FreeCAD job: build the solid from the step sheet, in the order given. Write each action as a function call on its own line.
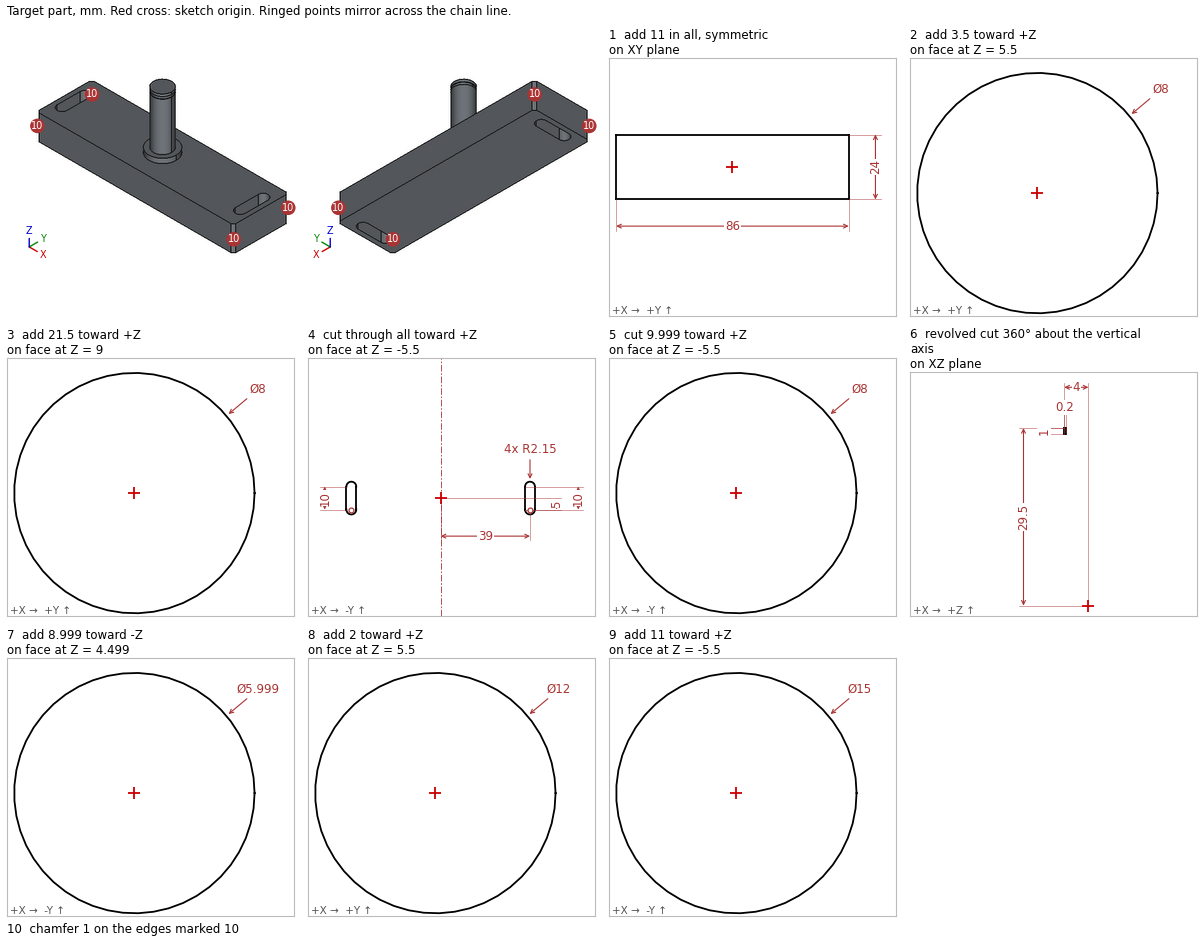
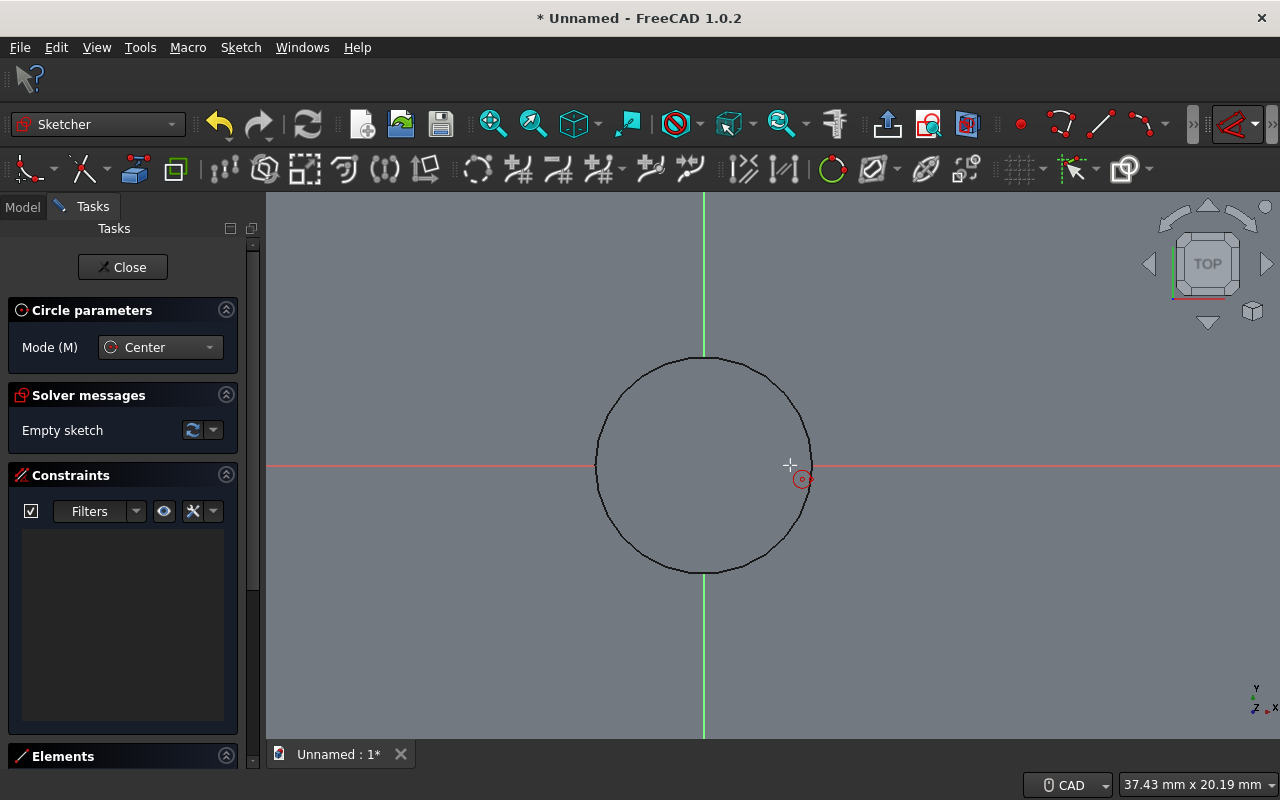
click(704, 465)
move(819, 351)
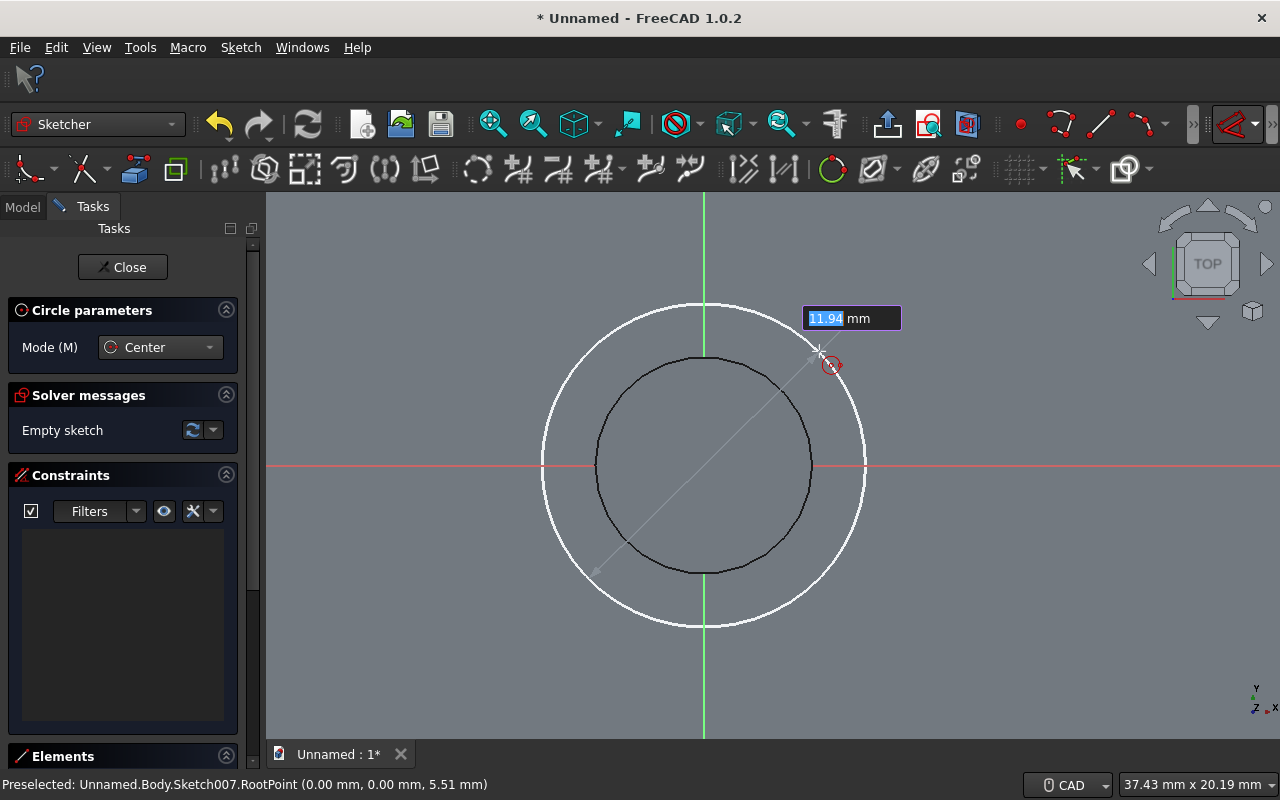
text(12)
key(Return)
key(Escape)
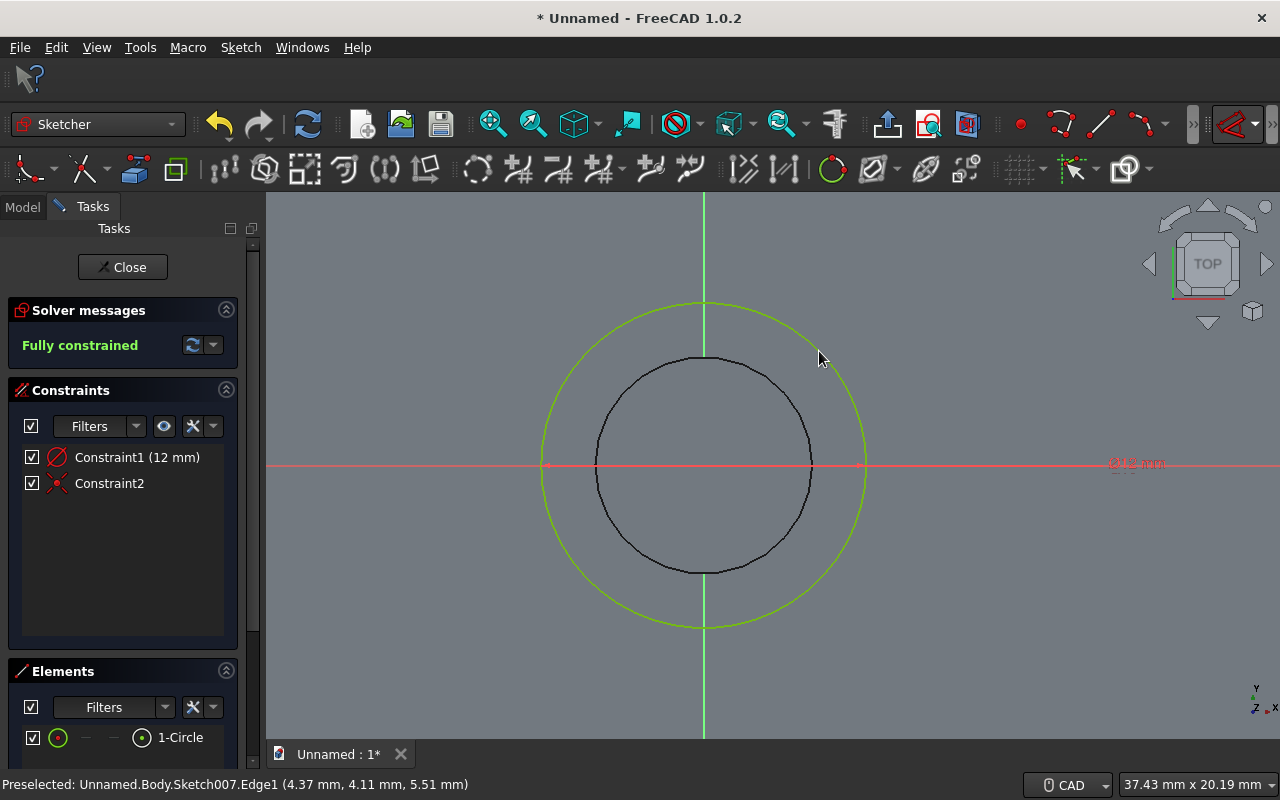
click(123, 267)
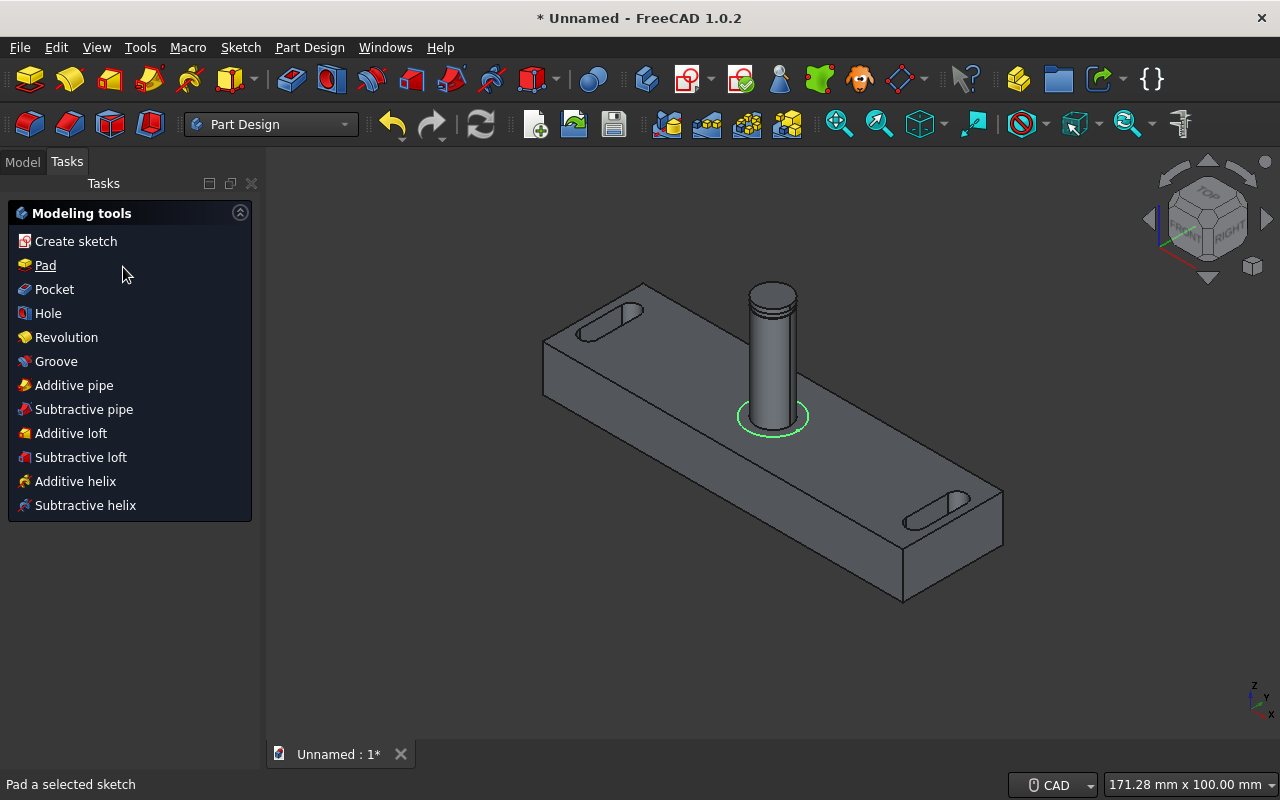
click(30, 80)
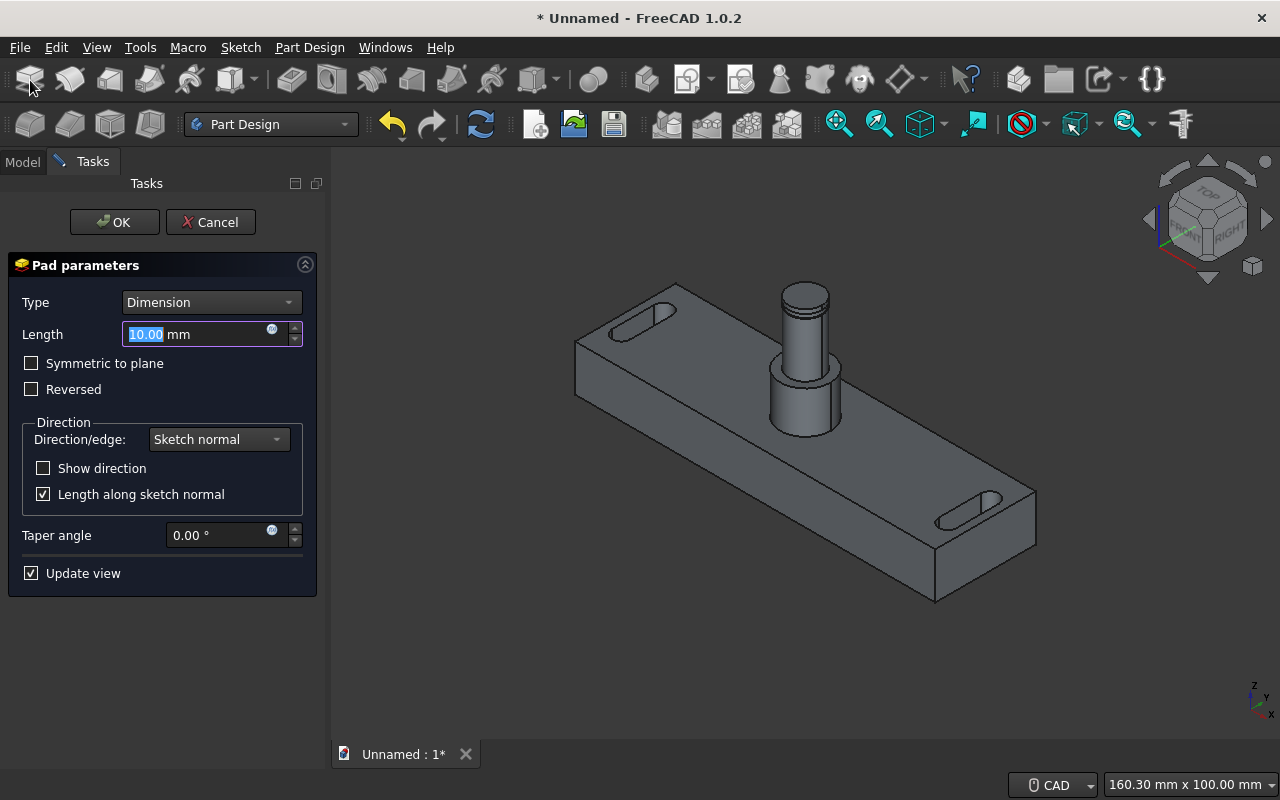
text(2)
key(Tab)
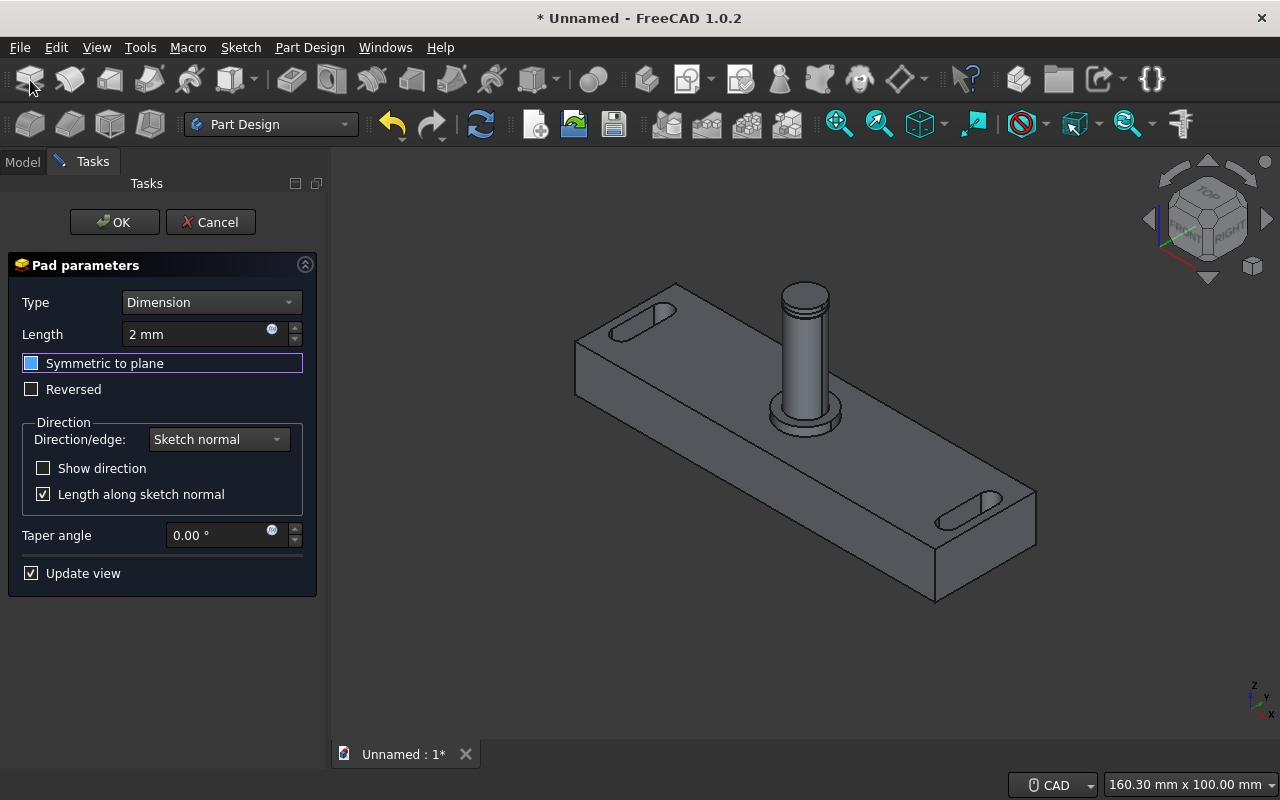
click(115, 222)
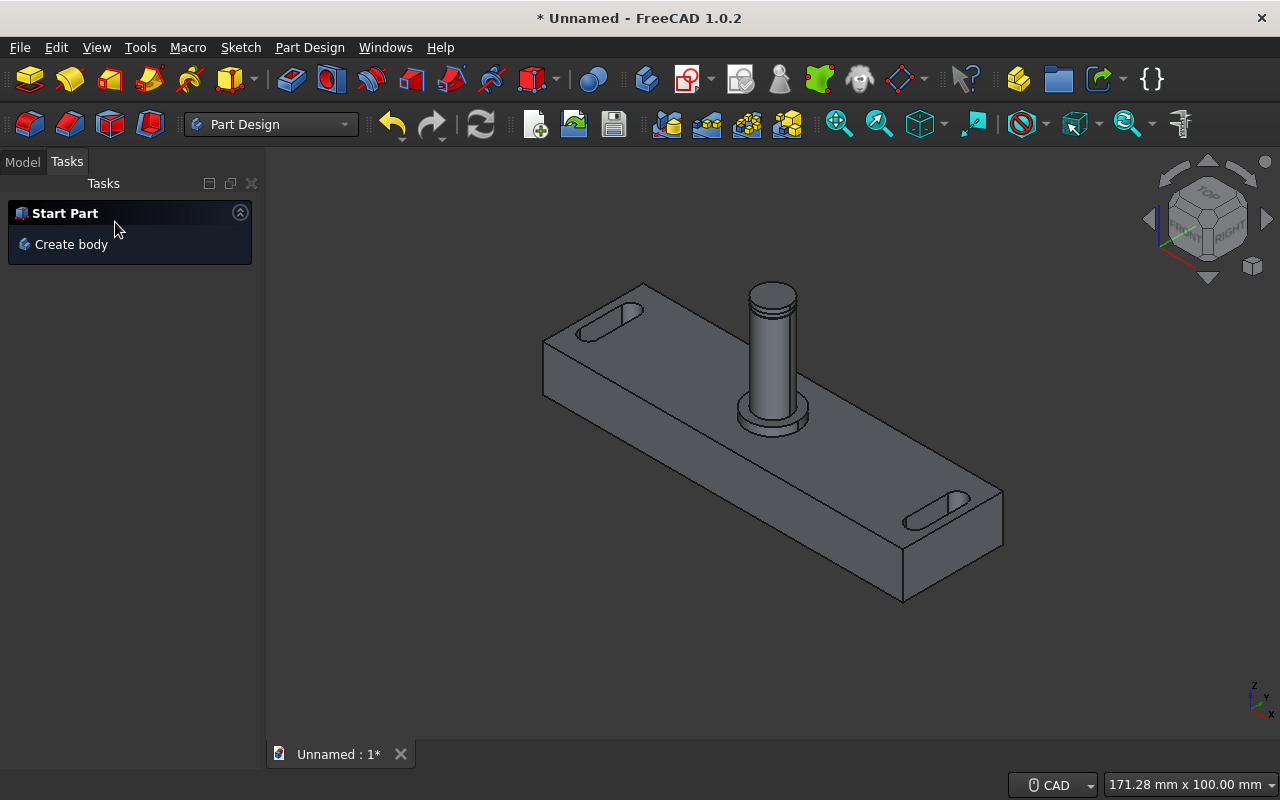
key(5)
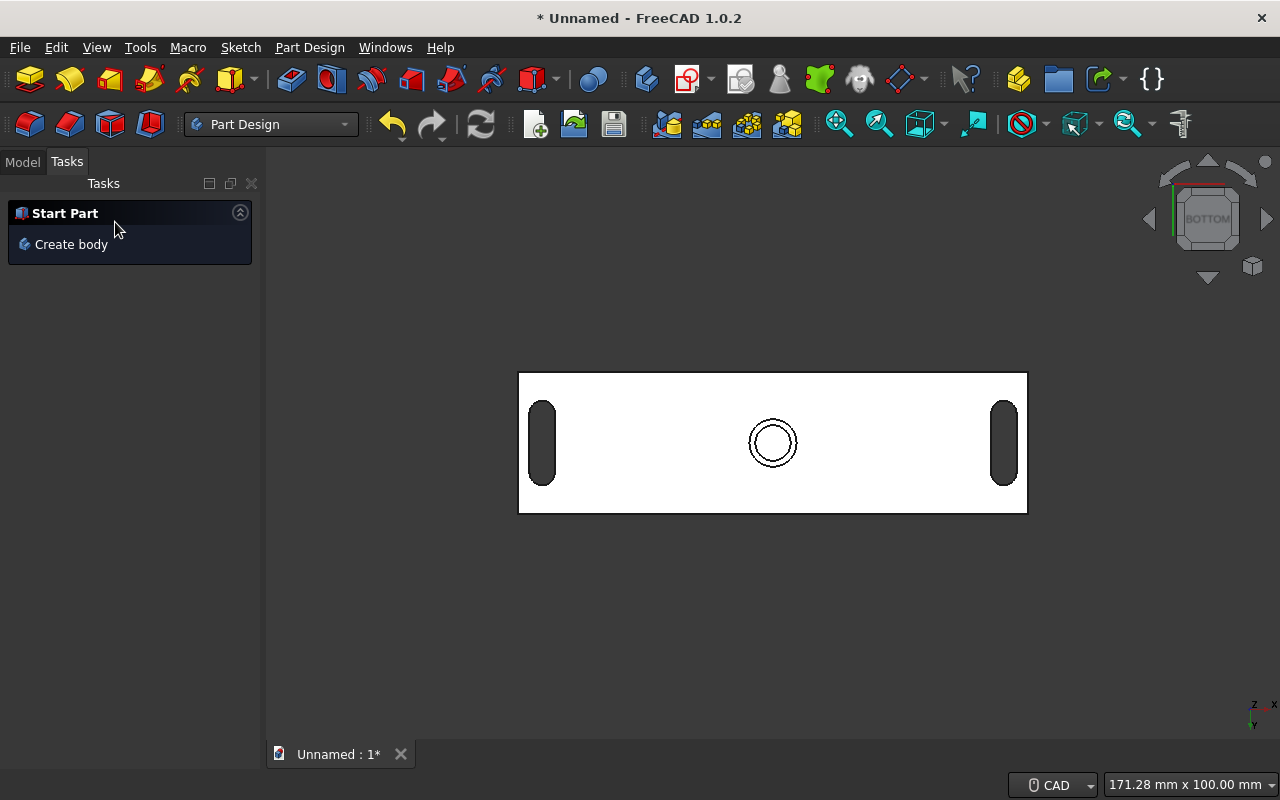
click(918, 442)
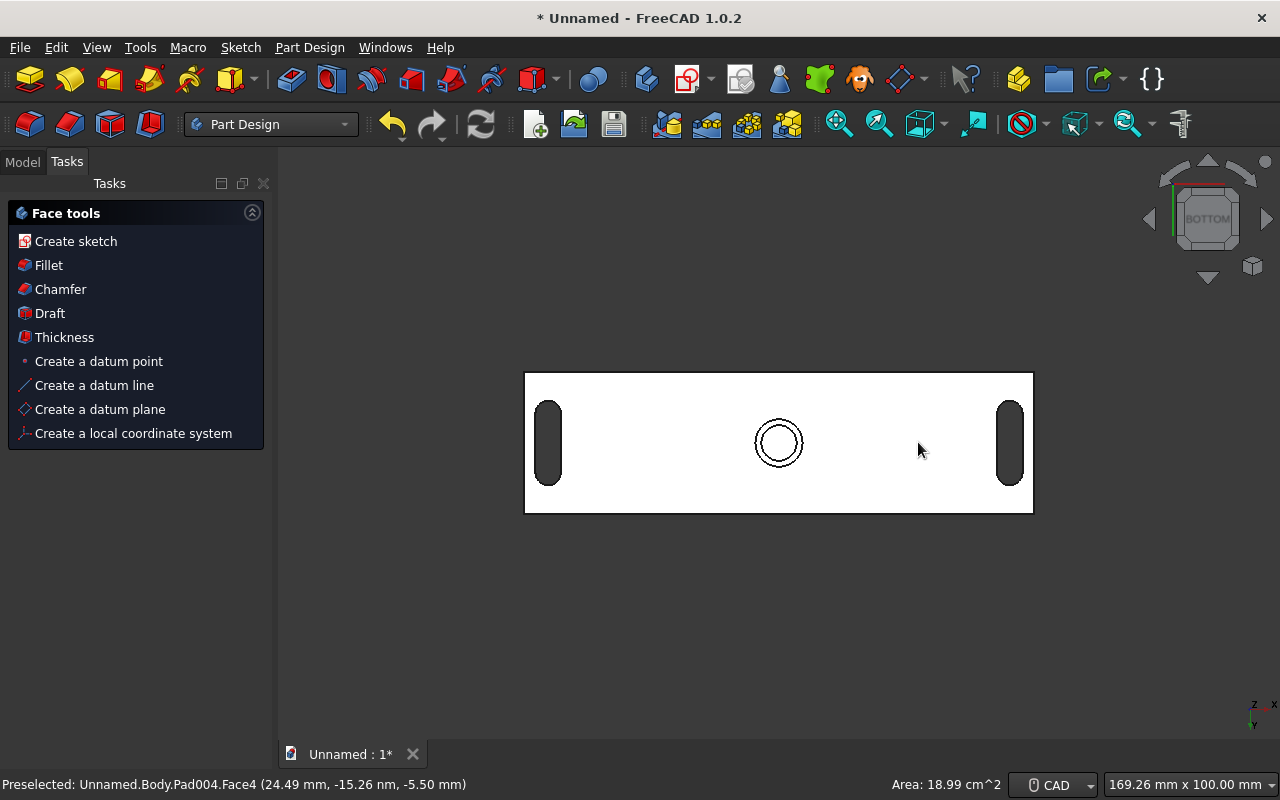
click(688, 80)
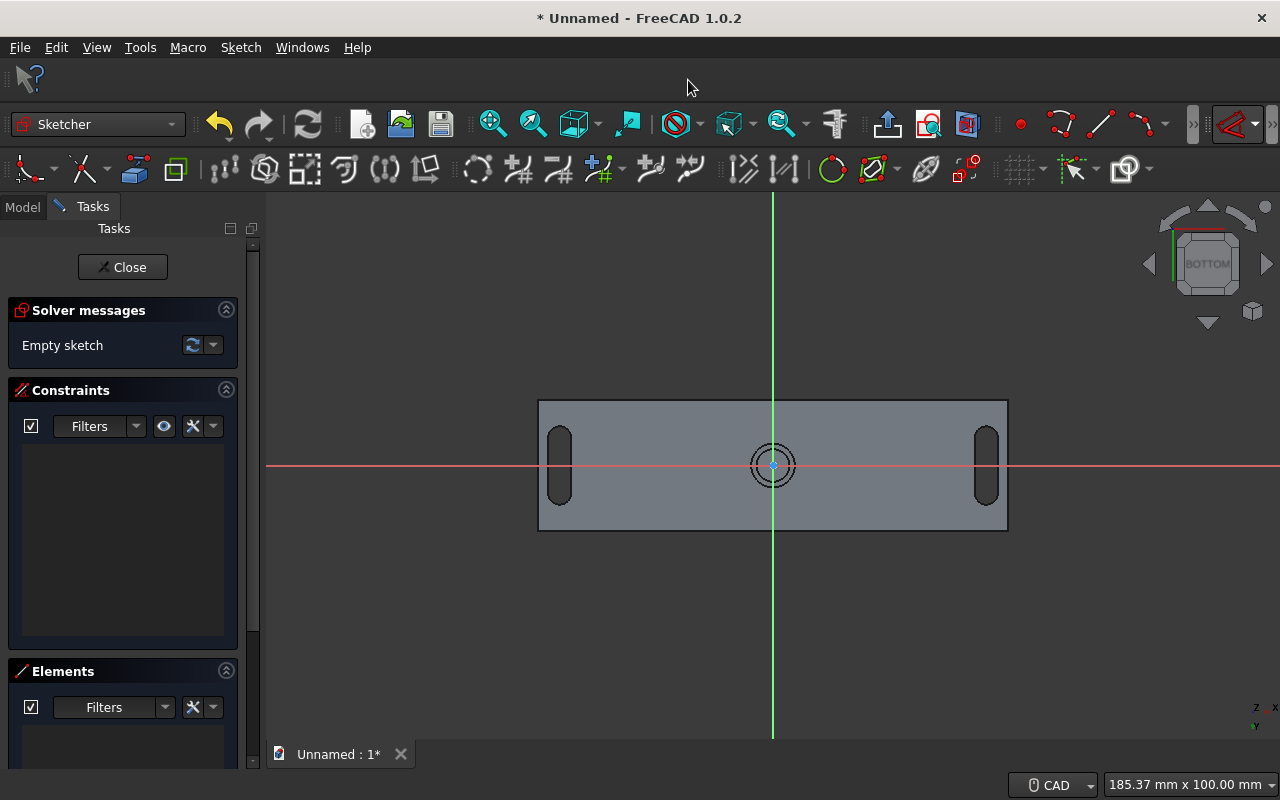
scroll(795, 466, up, 7)